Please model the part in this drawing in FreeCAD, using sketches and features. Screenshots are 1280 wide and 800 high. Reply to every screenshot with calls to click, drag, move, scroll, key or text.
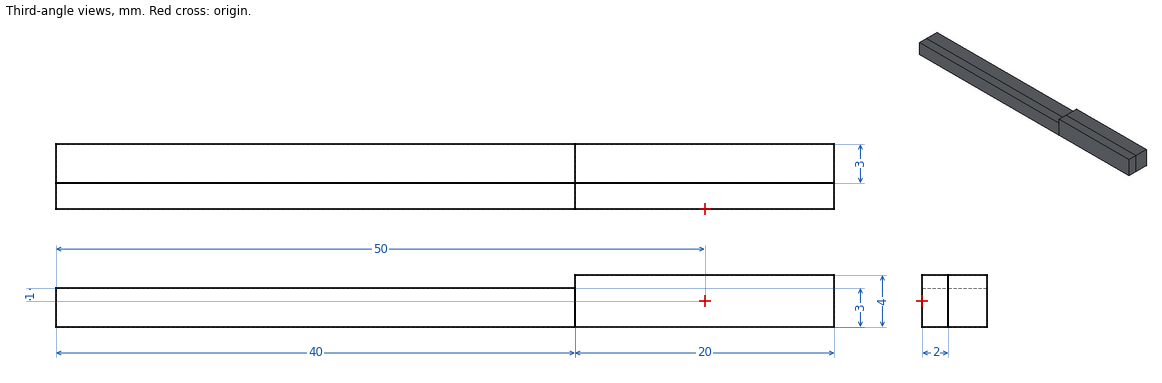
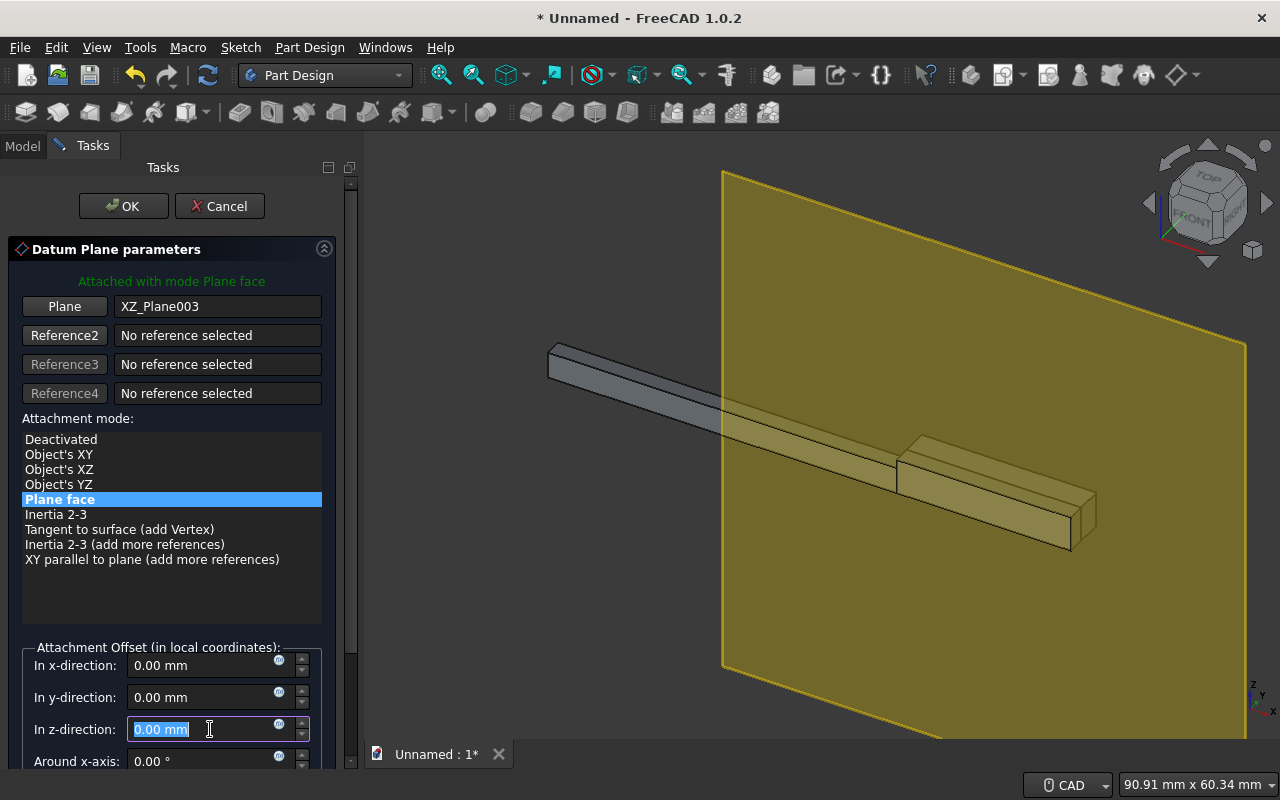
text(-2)
key(Tab)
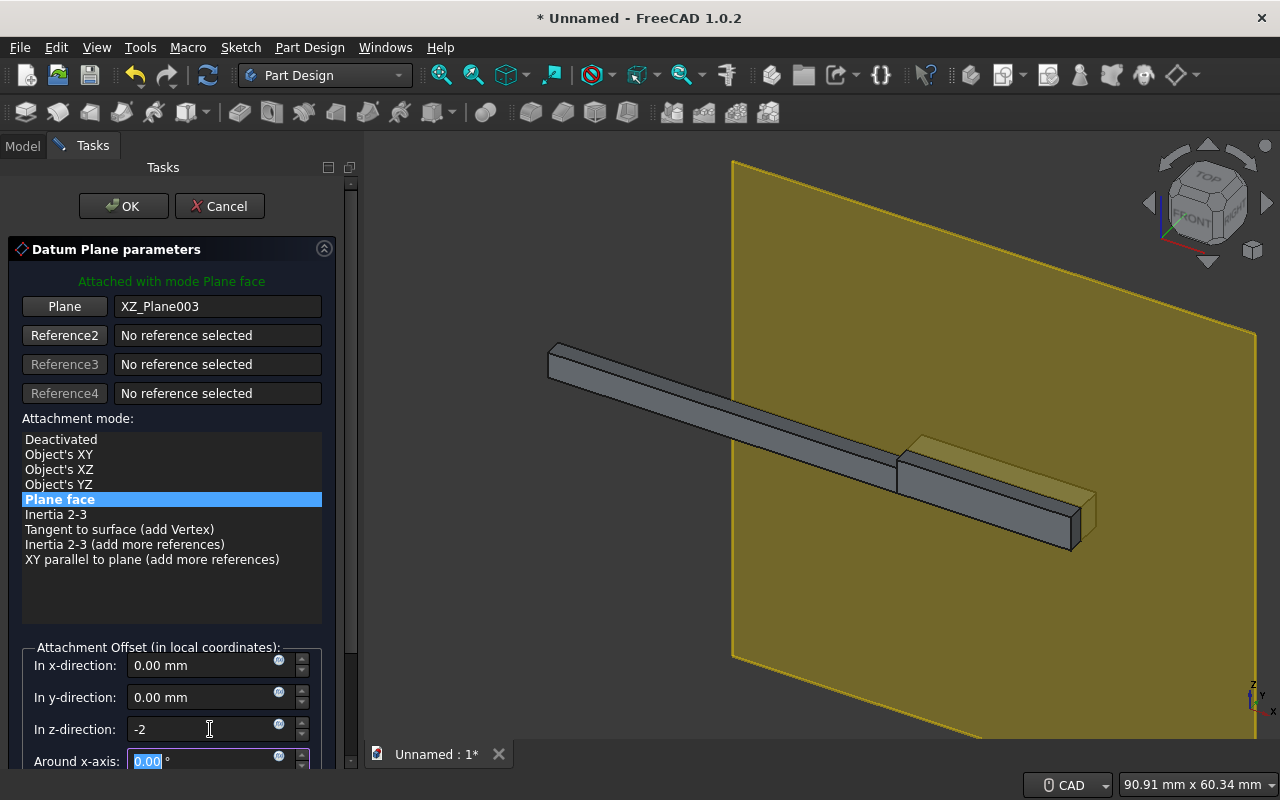
click(124, 206)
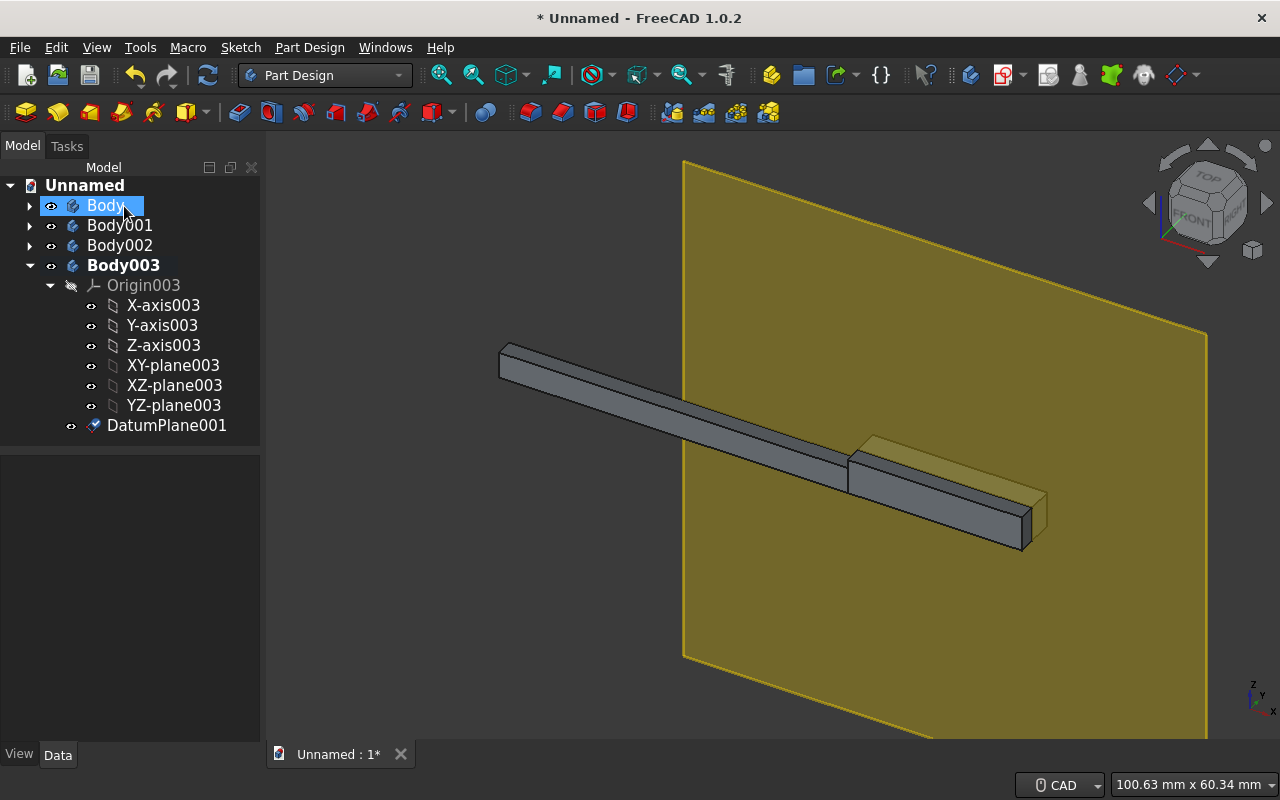
click(116, 426)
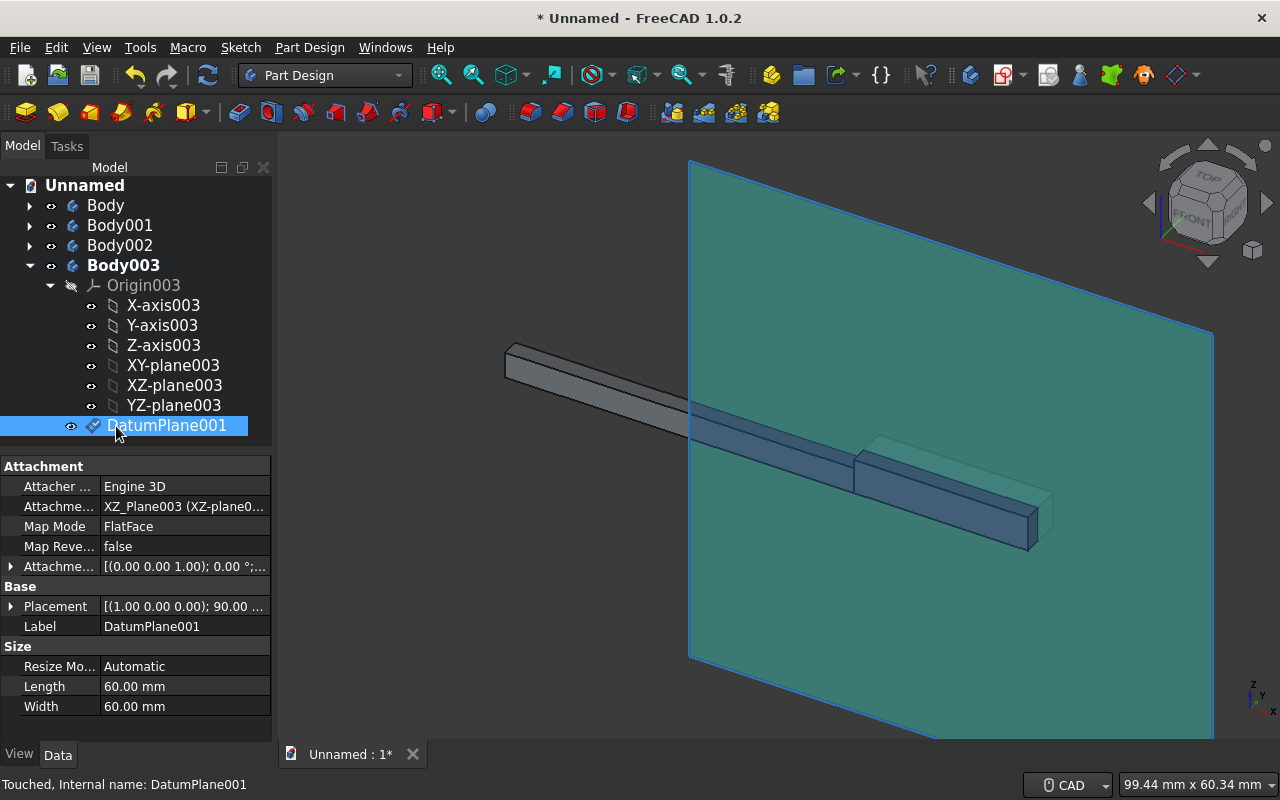
click(1004, 76)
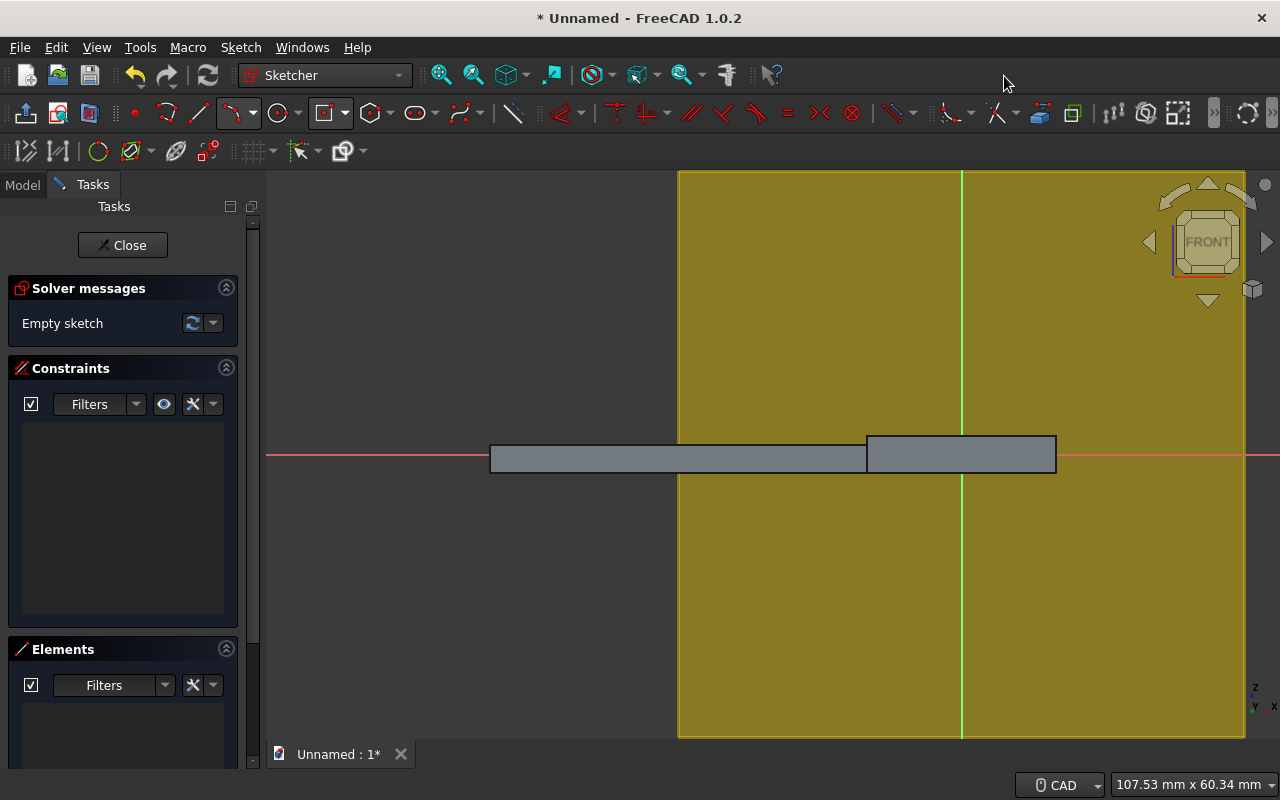
click(348, 114)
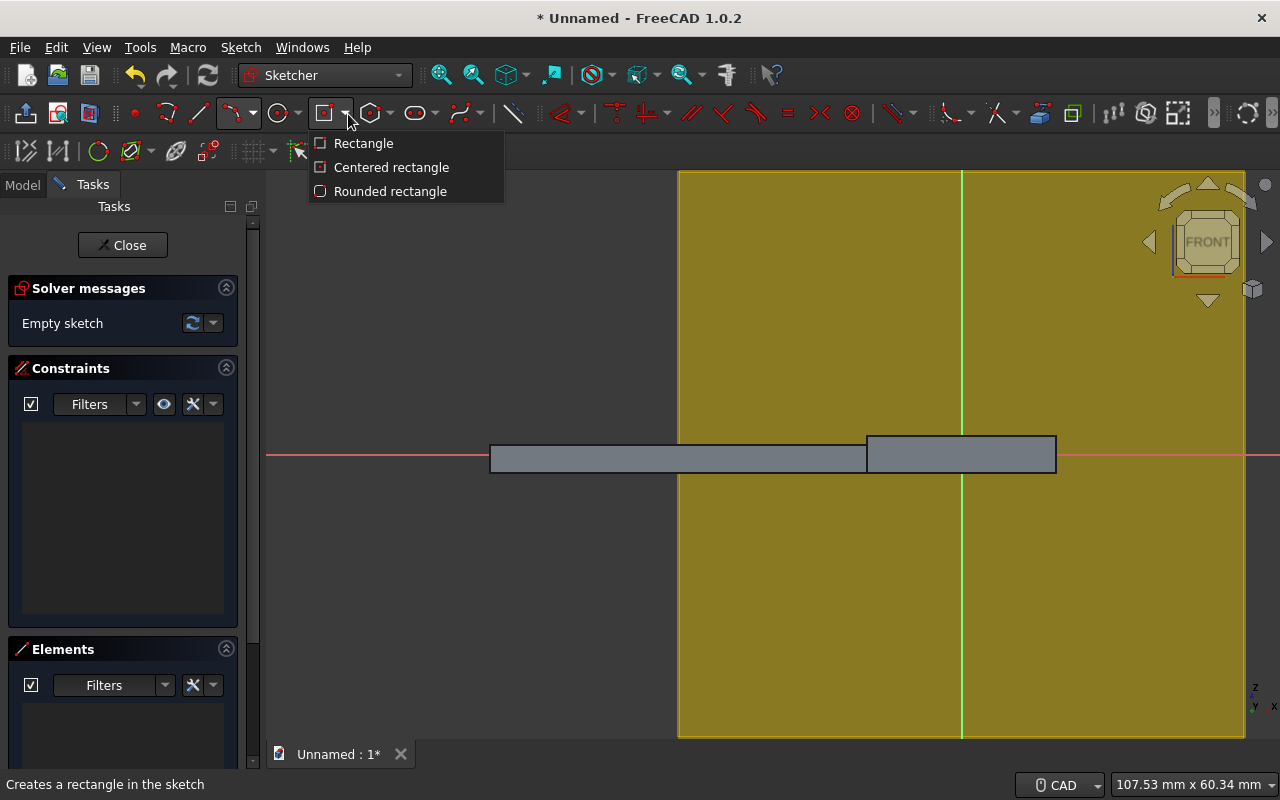
click(406, 143)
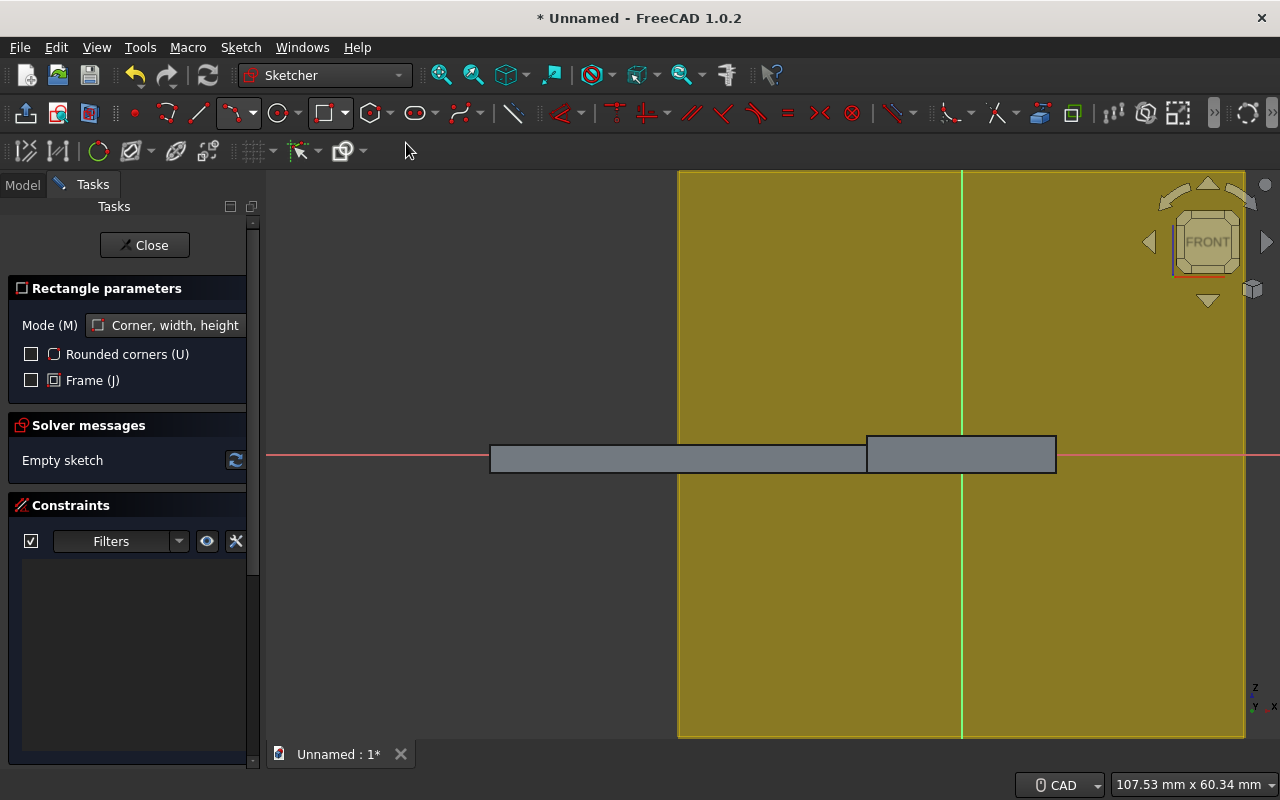
scroll(490, 445, up, 3)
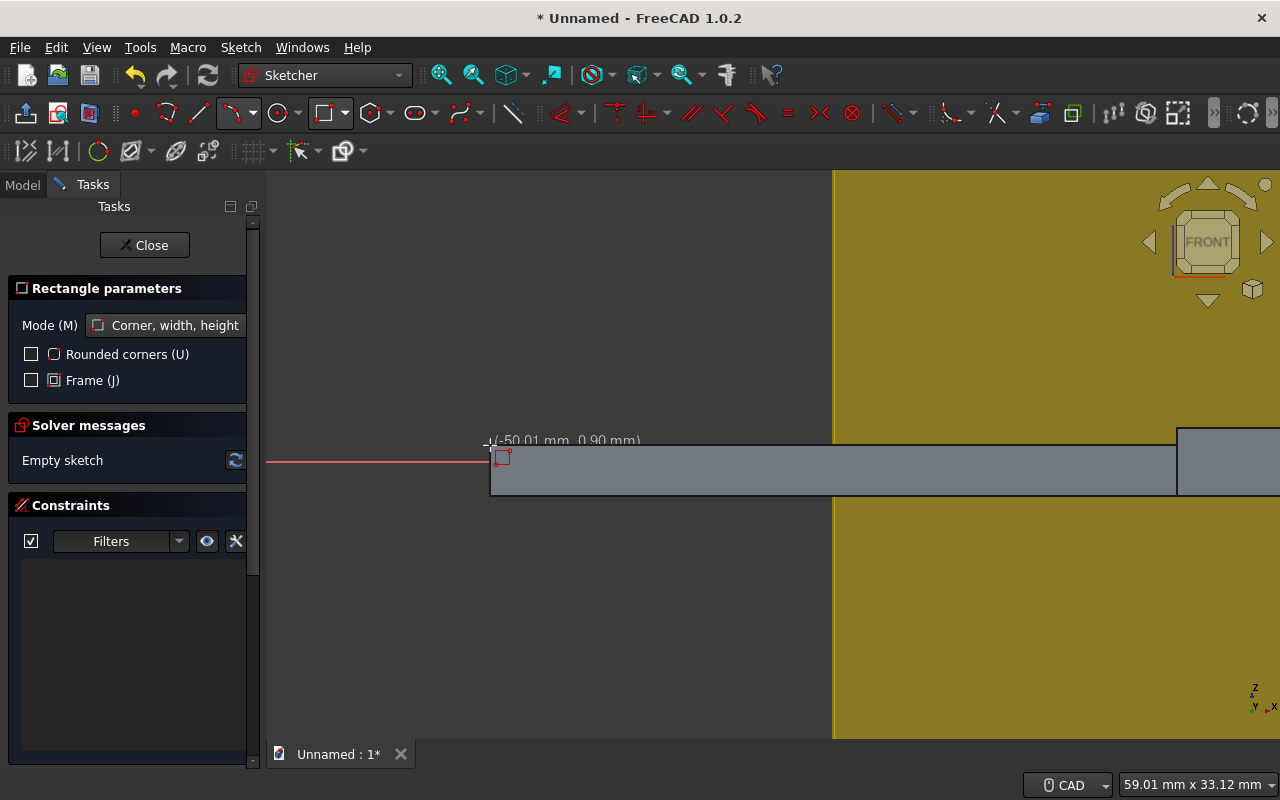
click(490, 445)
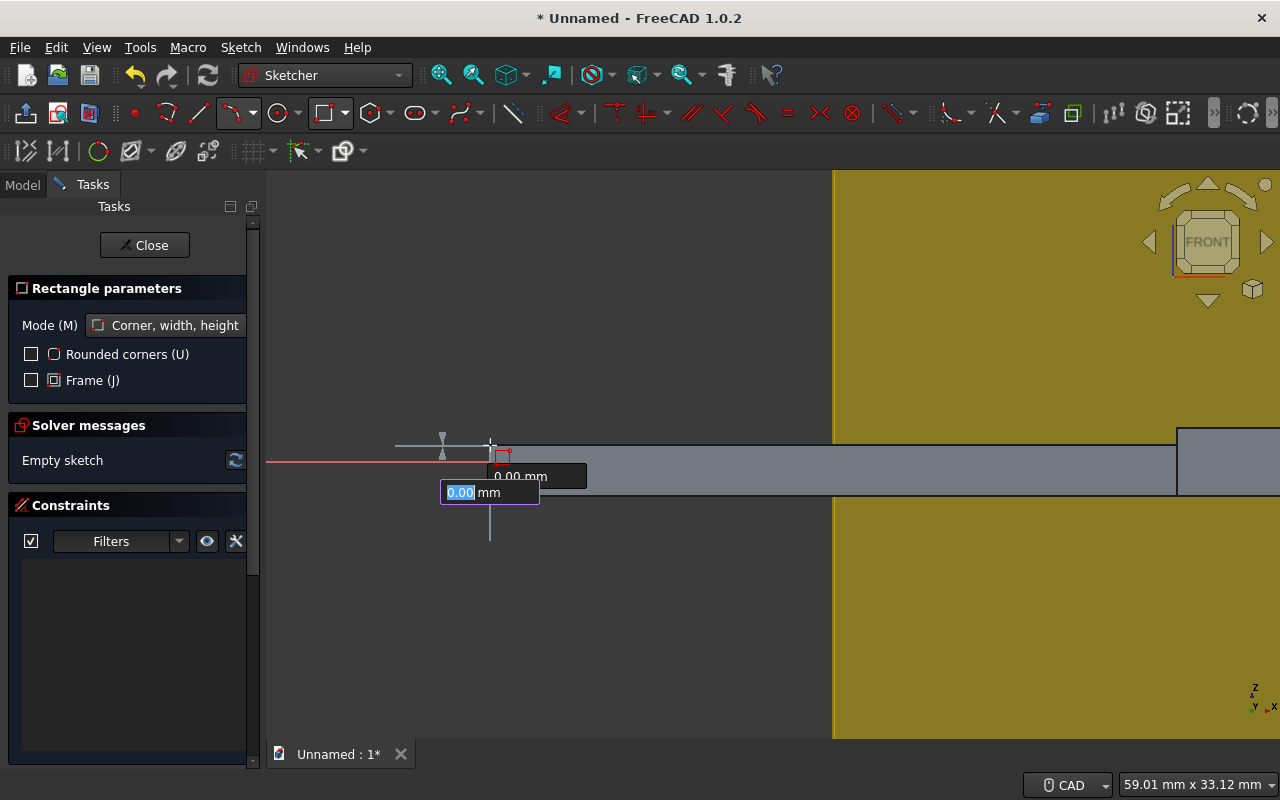
scroll(294, 422, down, 2)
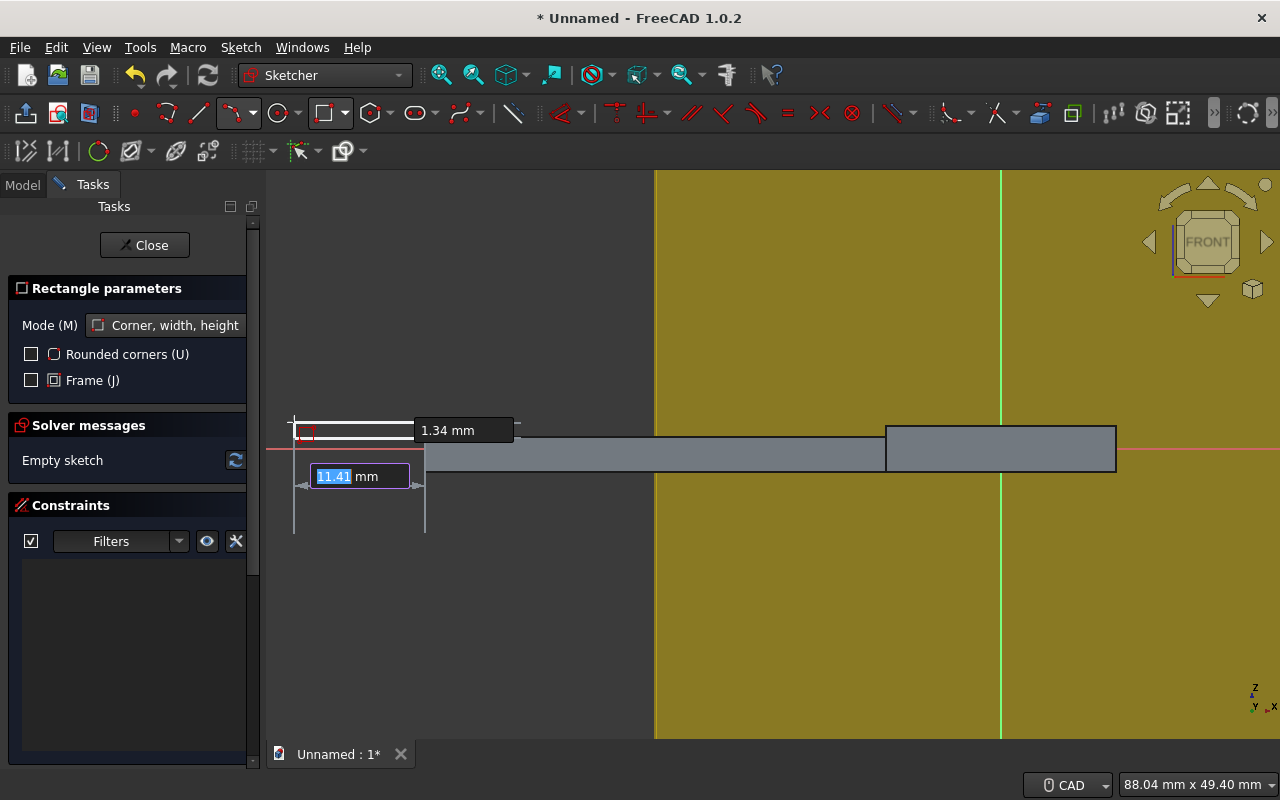
click(886, 472)
key(Escape)